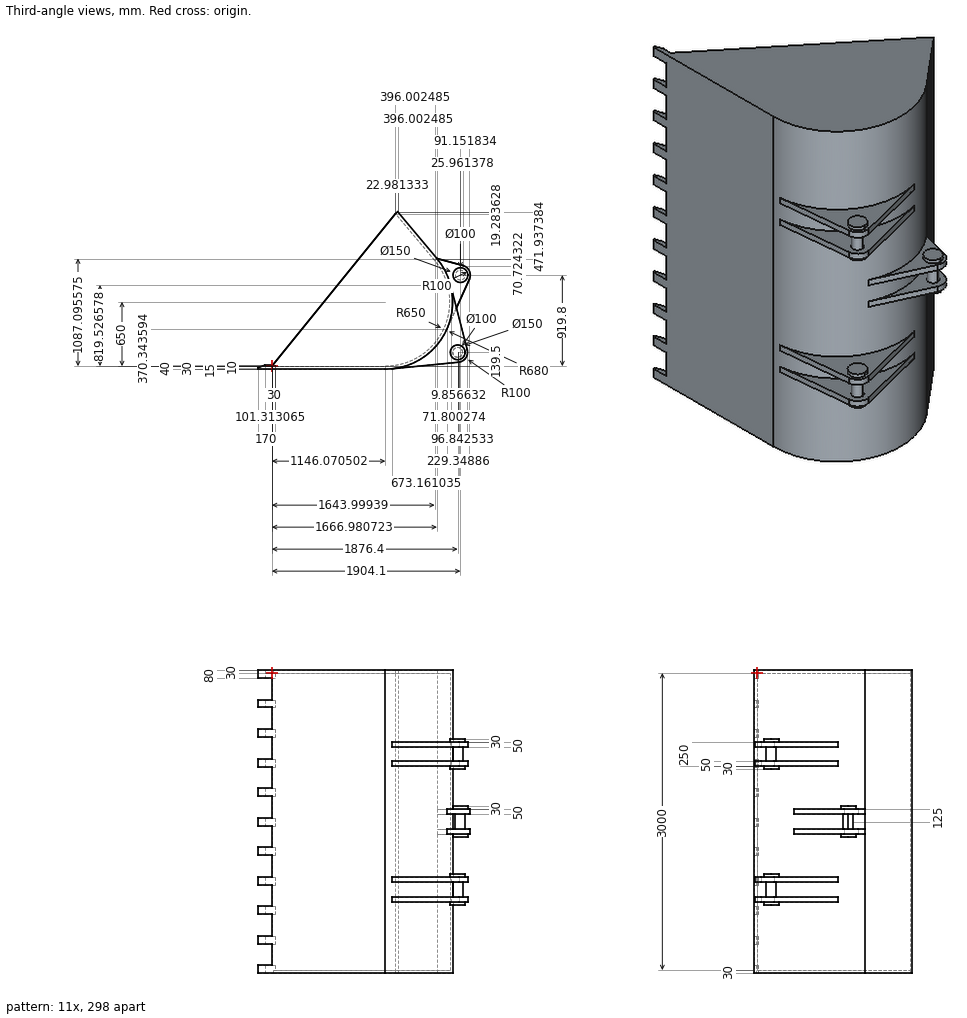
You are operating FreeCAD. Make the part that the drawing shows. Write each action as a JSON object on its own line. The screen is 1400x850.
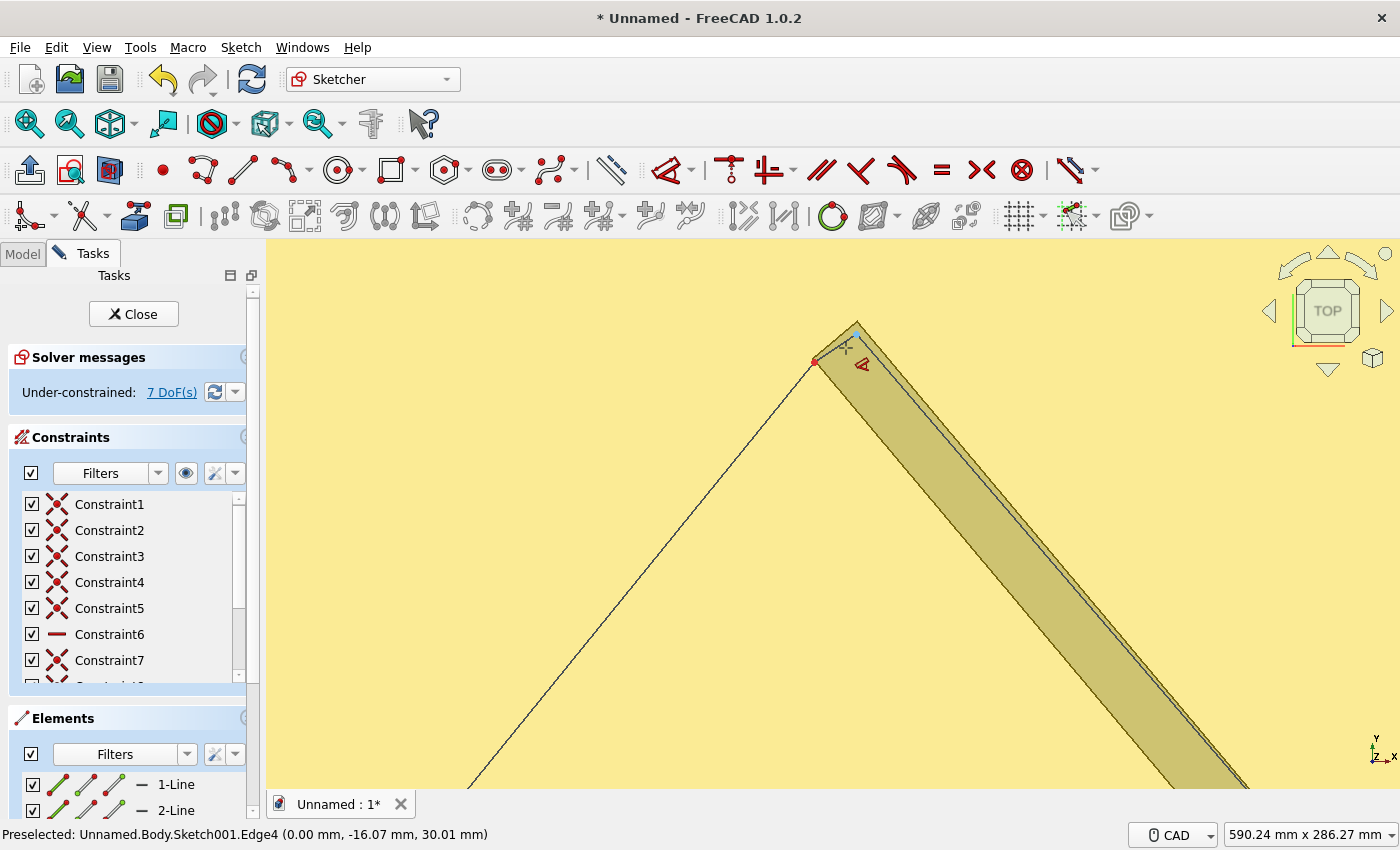
{"action": "left_click", "coordinate": [844, 343]}
{"action": "left_click", "coordinate": [836, 300]}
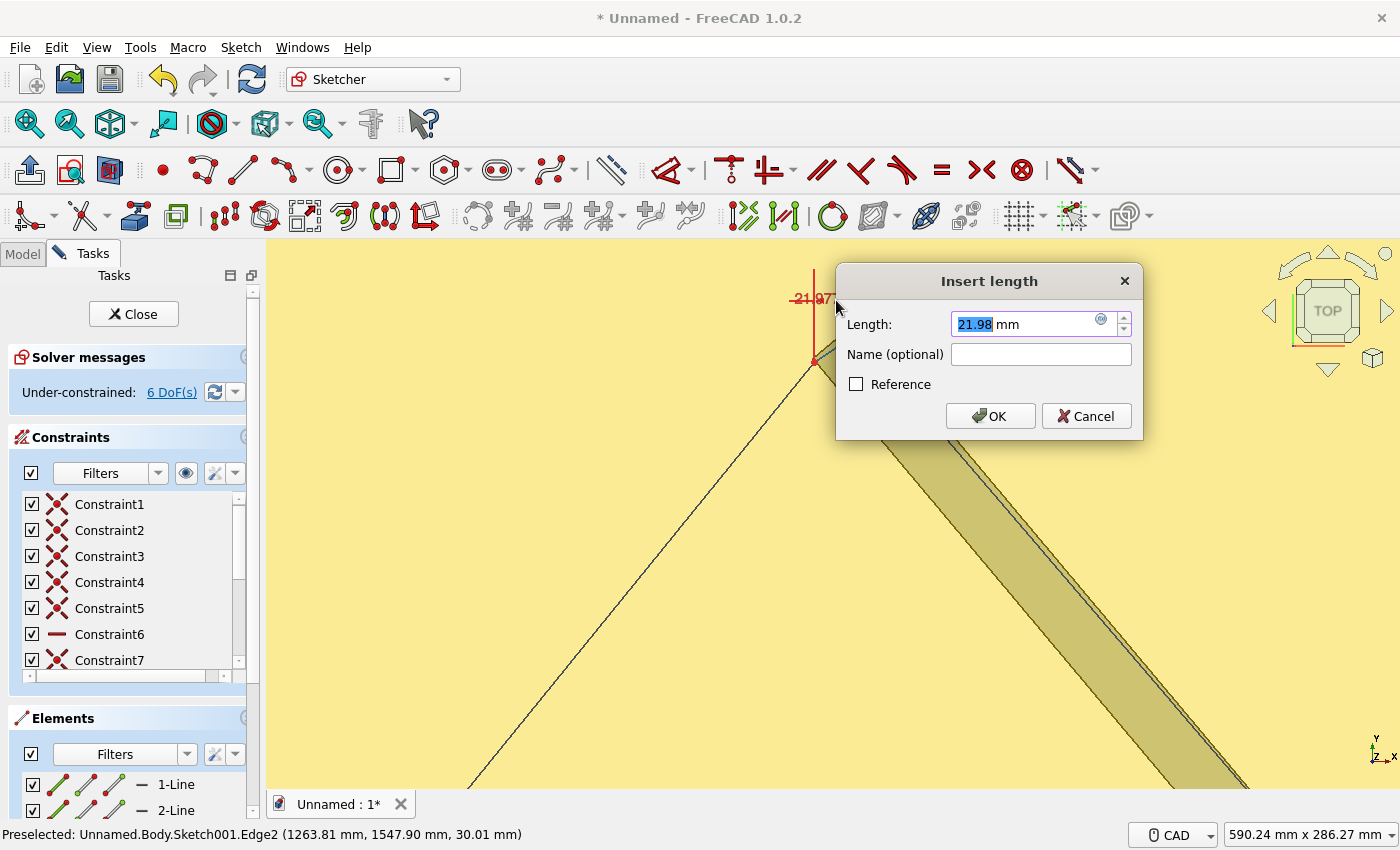
{"action": "type", "text": "22.981333"}
{"action": "key", "text": "Return"}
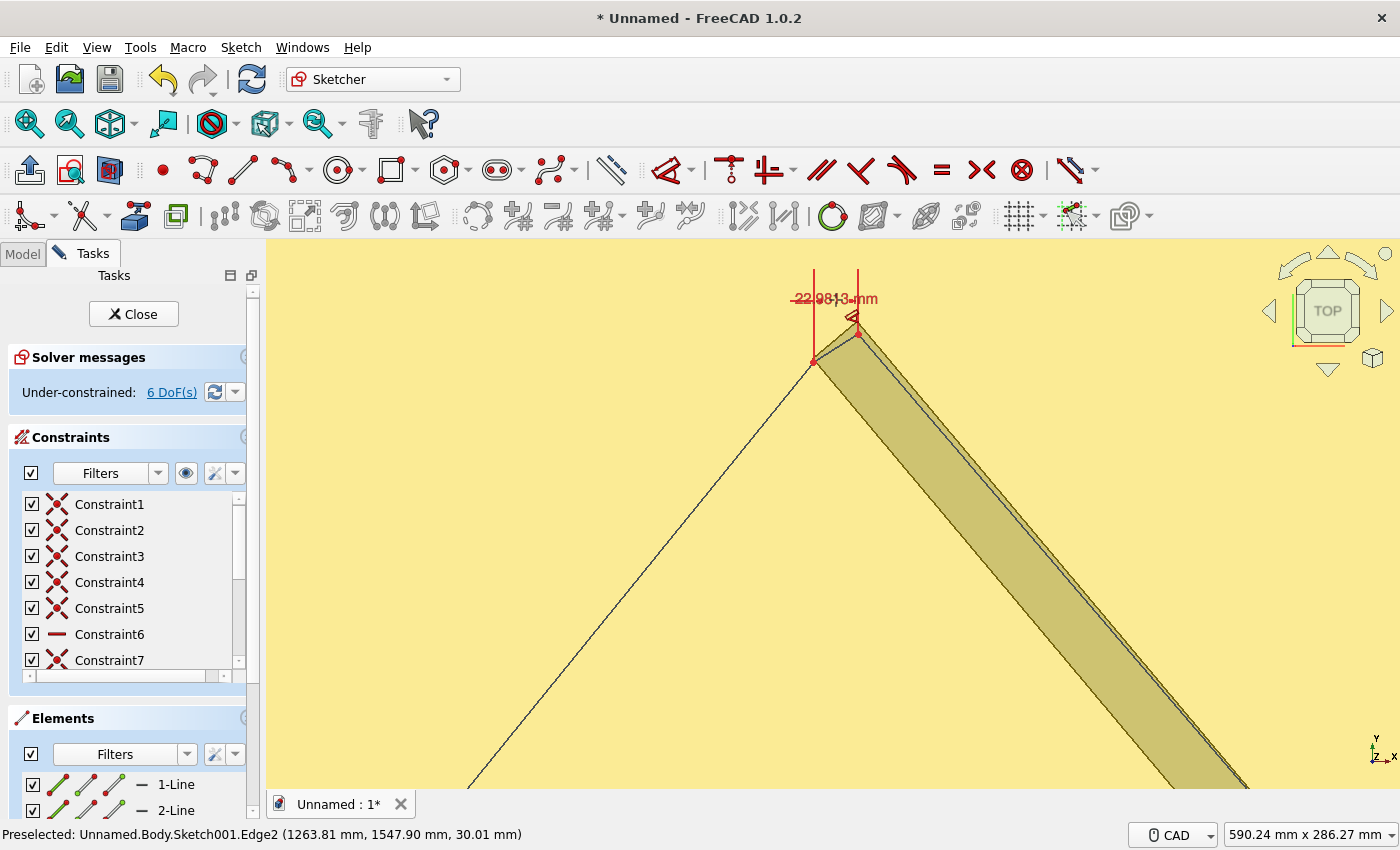
{"action": "left_click", "coordinate": [845, 343]}
{"action": "left_click", "coordinate": [892, 348]}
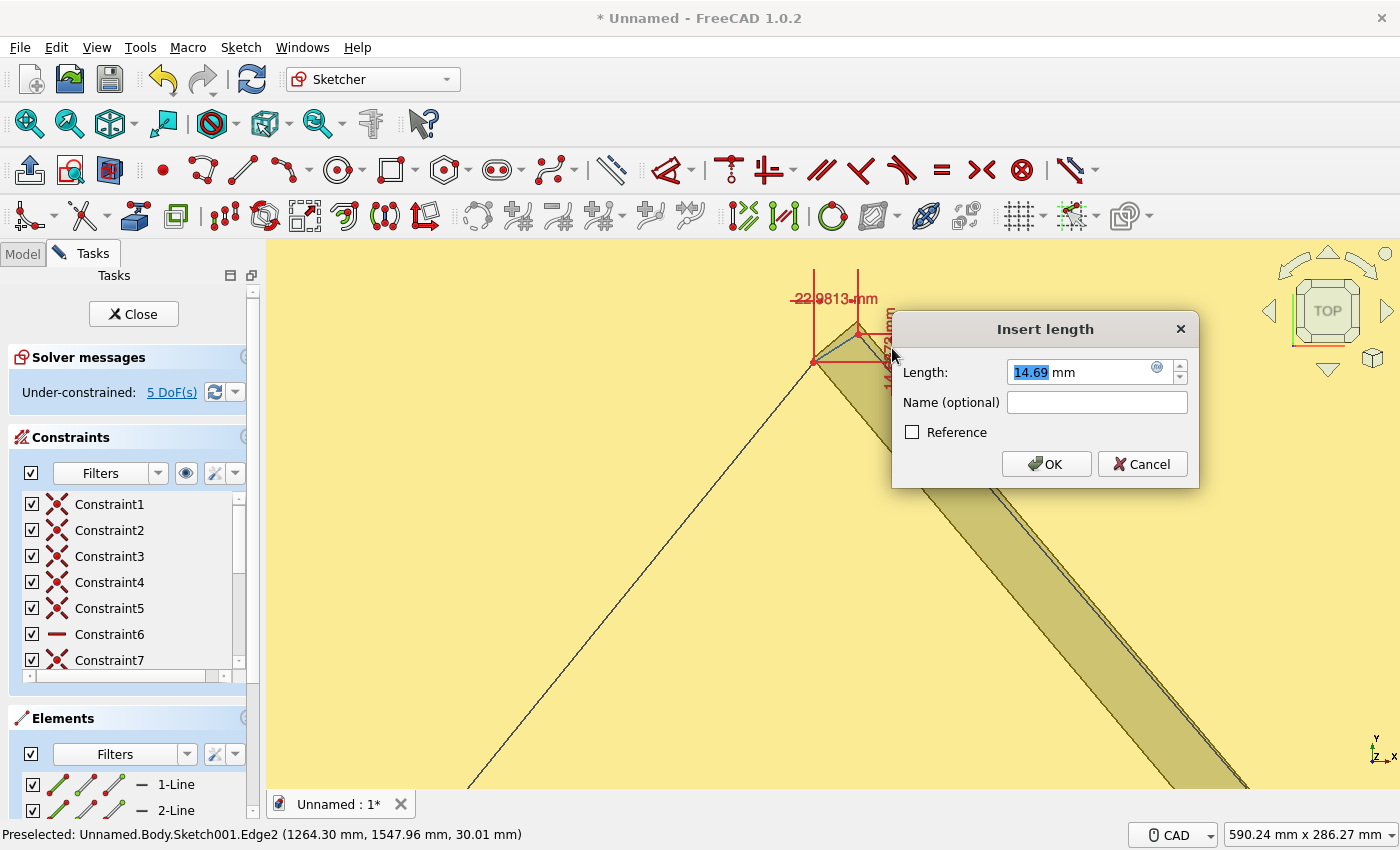
{"action": "type", "text": "19.283628"}
{"action": "key", "text": "Return"}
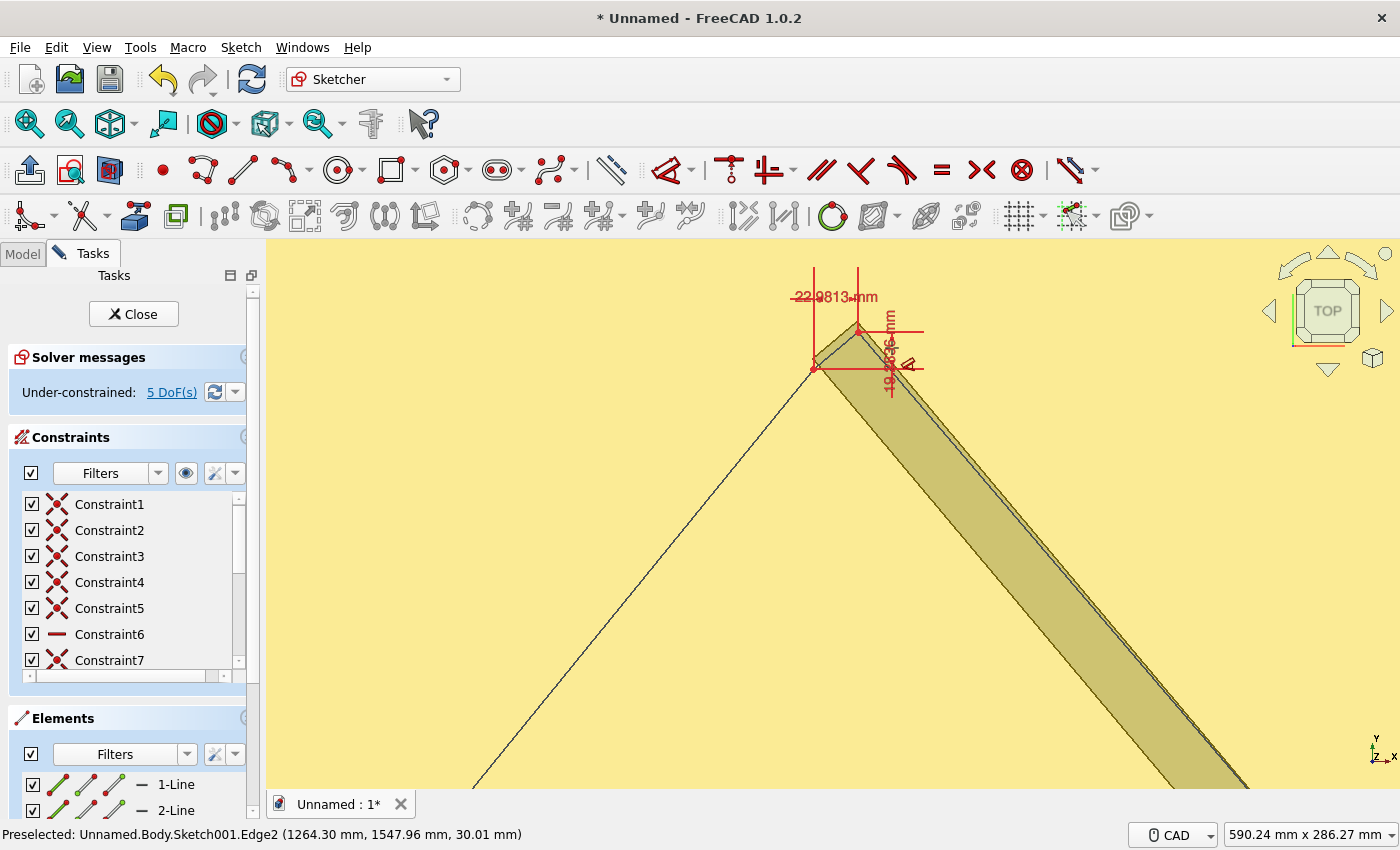
{"action": "scroll", "coordinate": [846, 348], "scroll_direction": "down", "scroll_amount": 11}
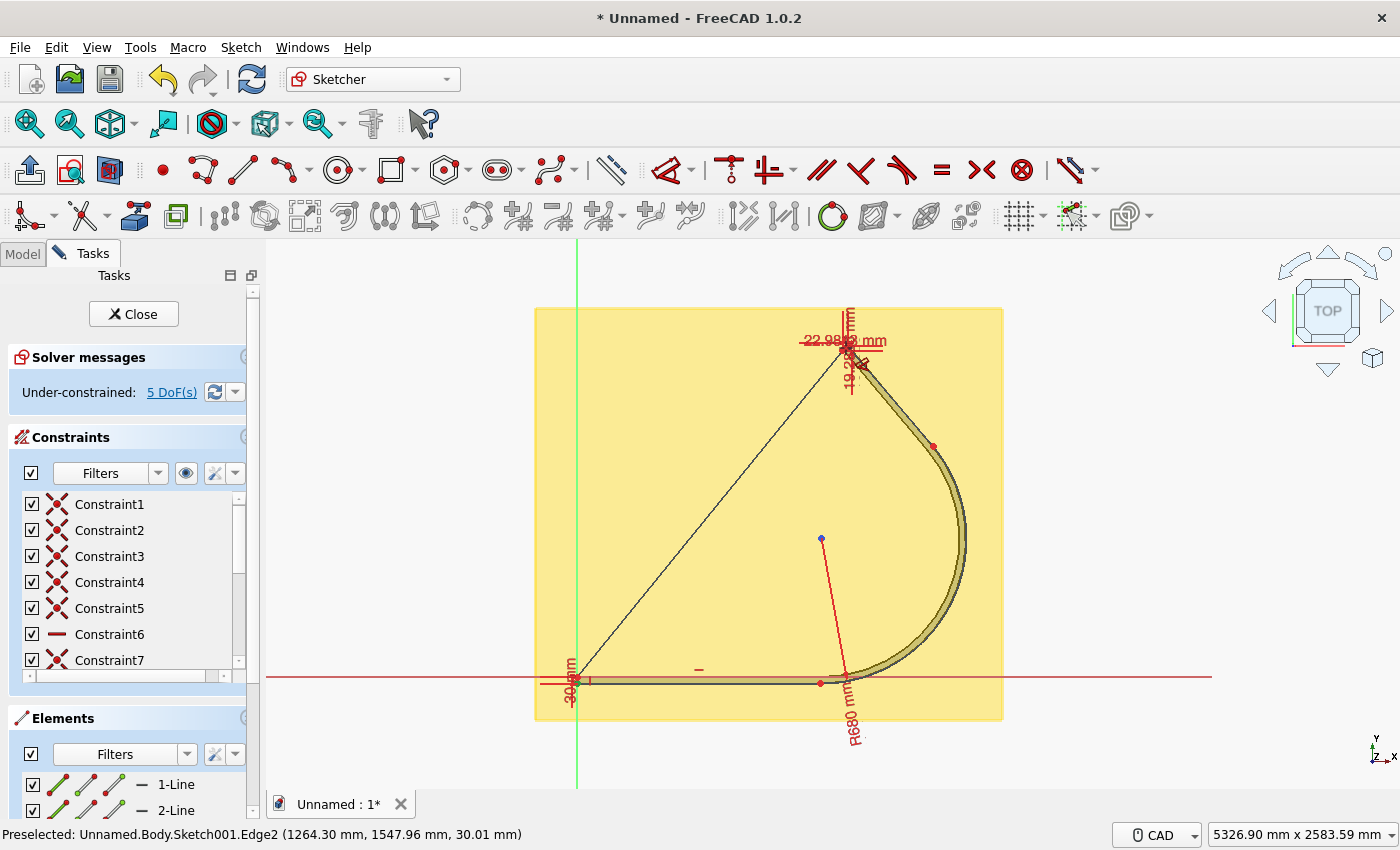
{"action": "scroll", "coordinate": [650, 684], "scroll_direction": "up", "scroll_amount": 4}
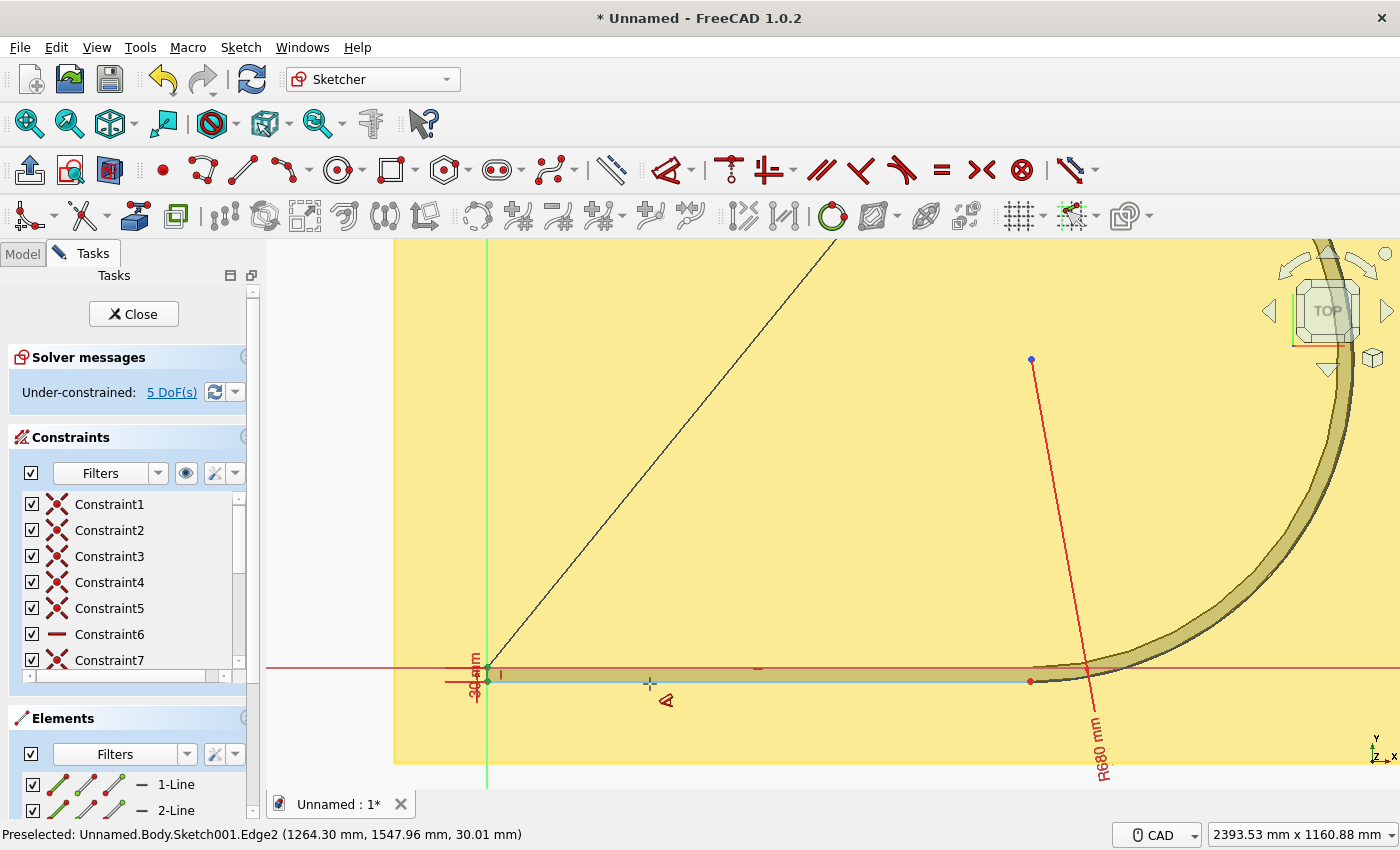
{"action": "left_click", "coordinate": [650, 682]}
{"action": "left_click", "coordinate": [759, 716]}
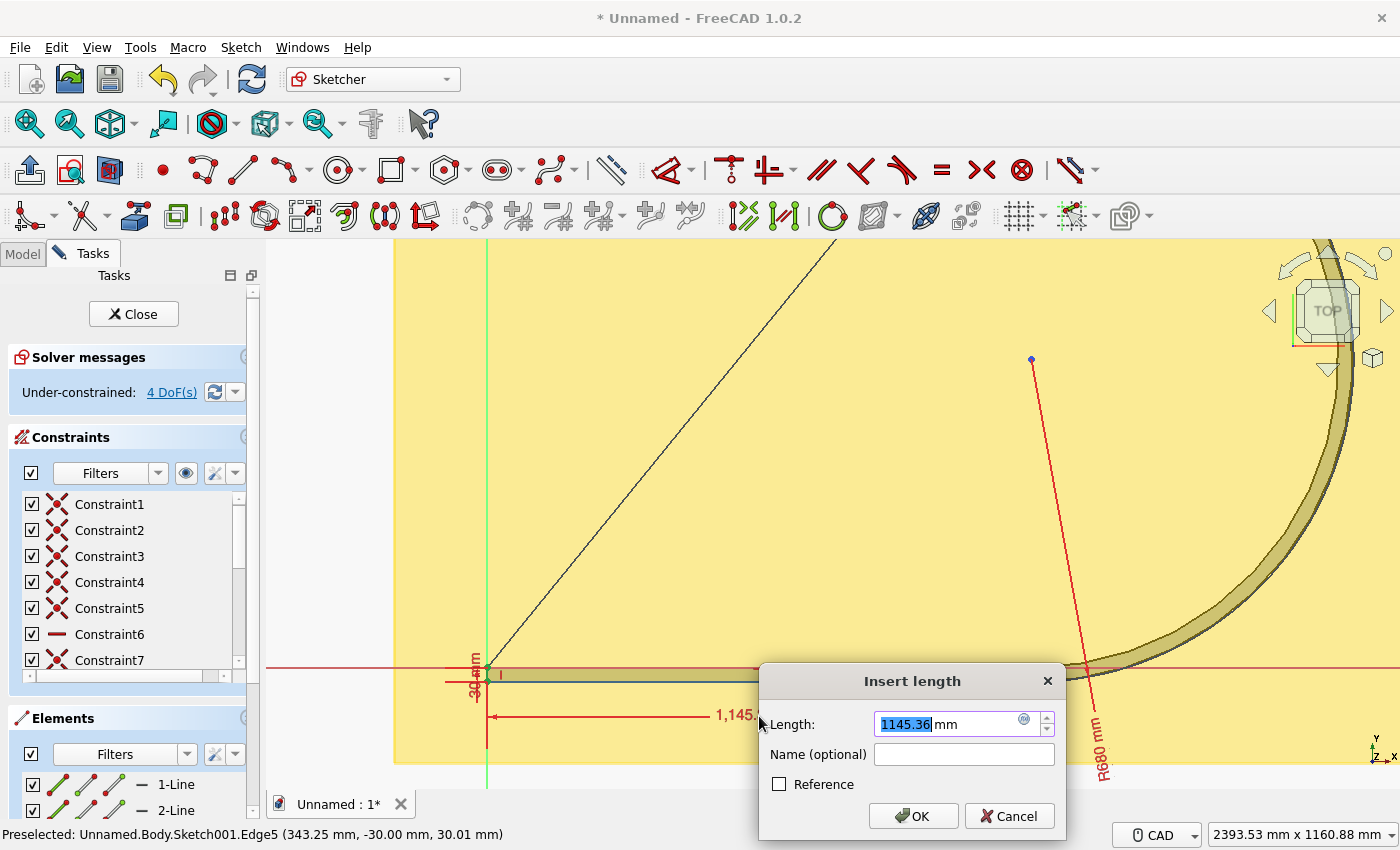
{"action": "type", "text": "1146.070502"}
{"action": "key", "text": "Return"}